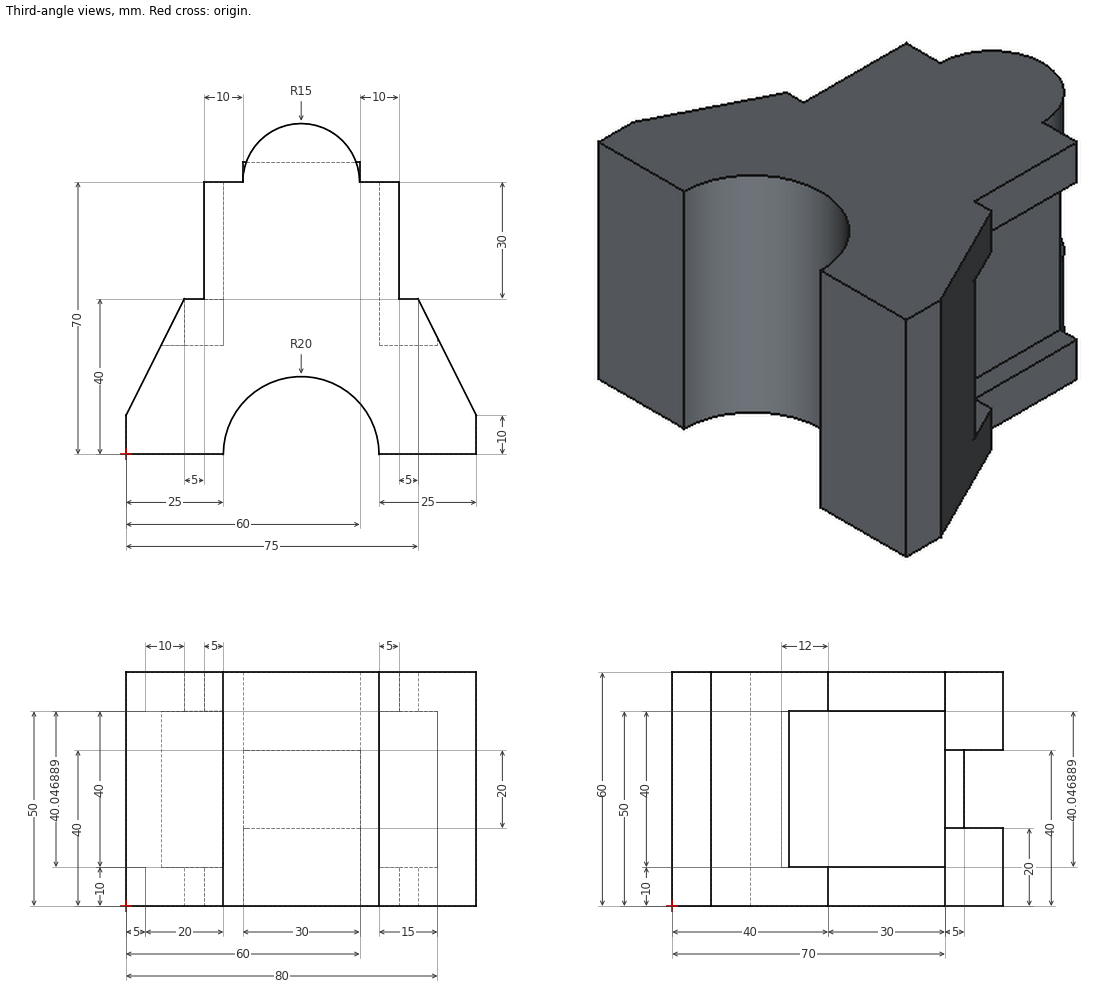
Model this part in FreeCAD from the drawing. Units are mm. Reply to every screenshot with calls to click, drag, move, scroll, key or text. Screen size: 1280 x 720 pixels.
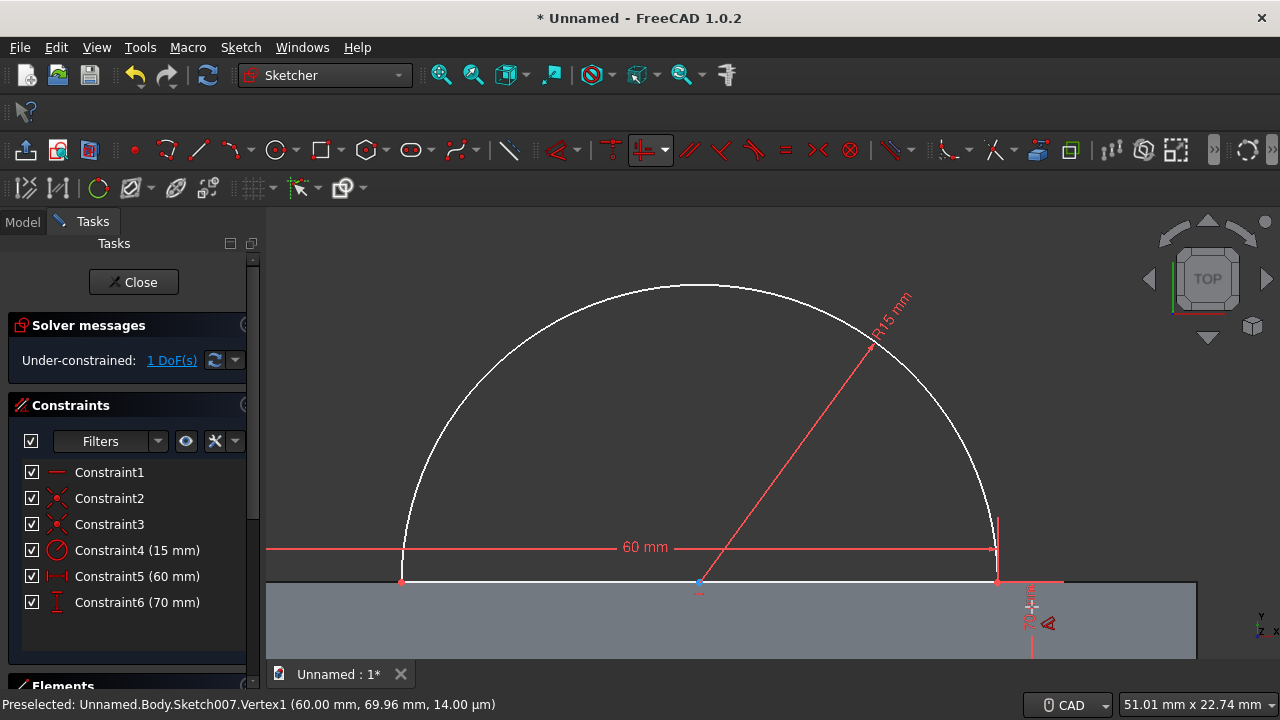
click(700, 583)
click(734, 607)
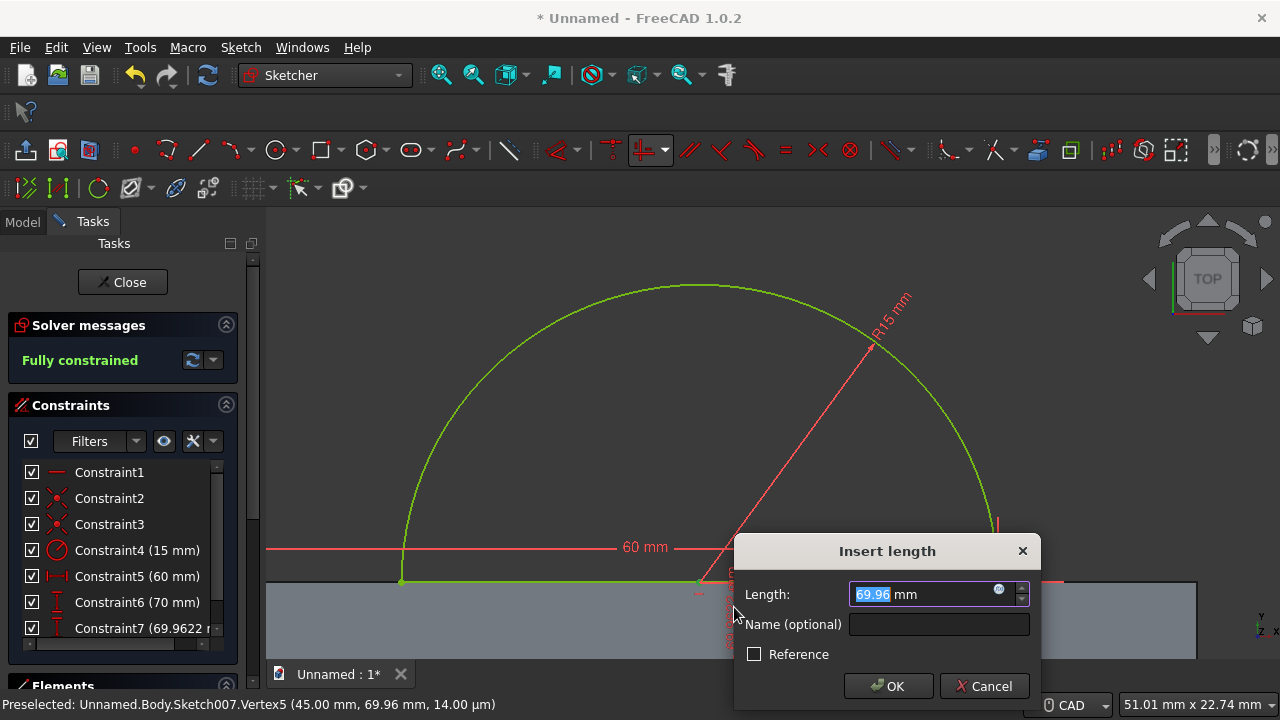
text(70)
key(Return)
key(Escape)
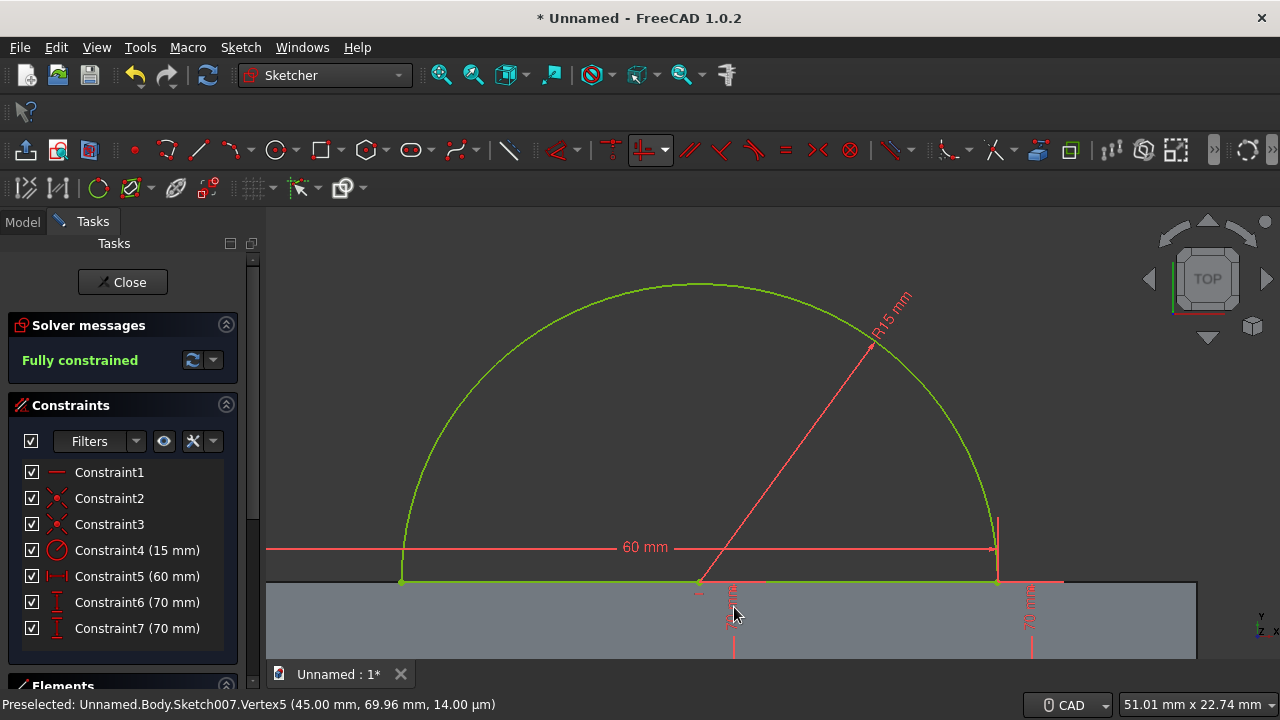
click(123, 282)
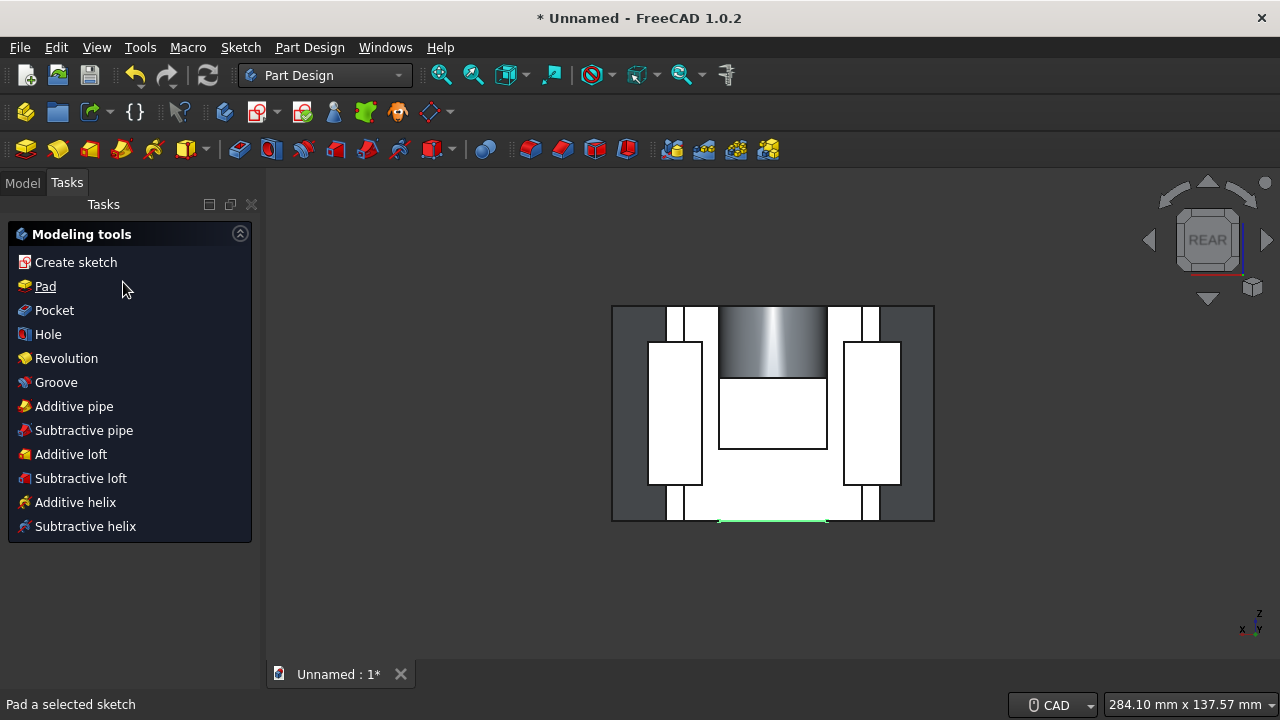
click(26, 150)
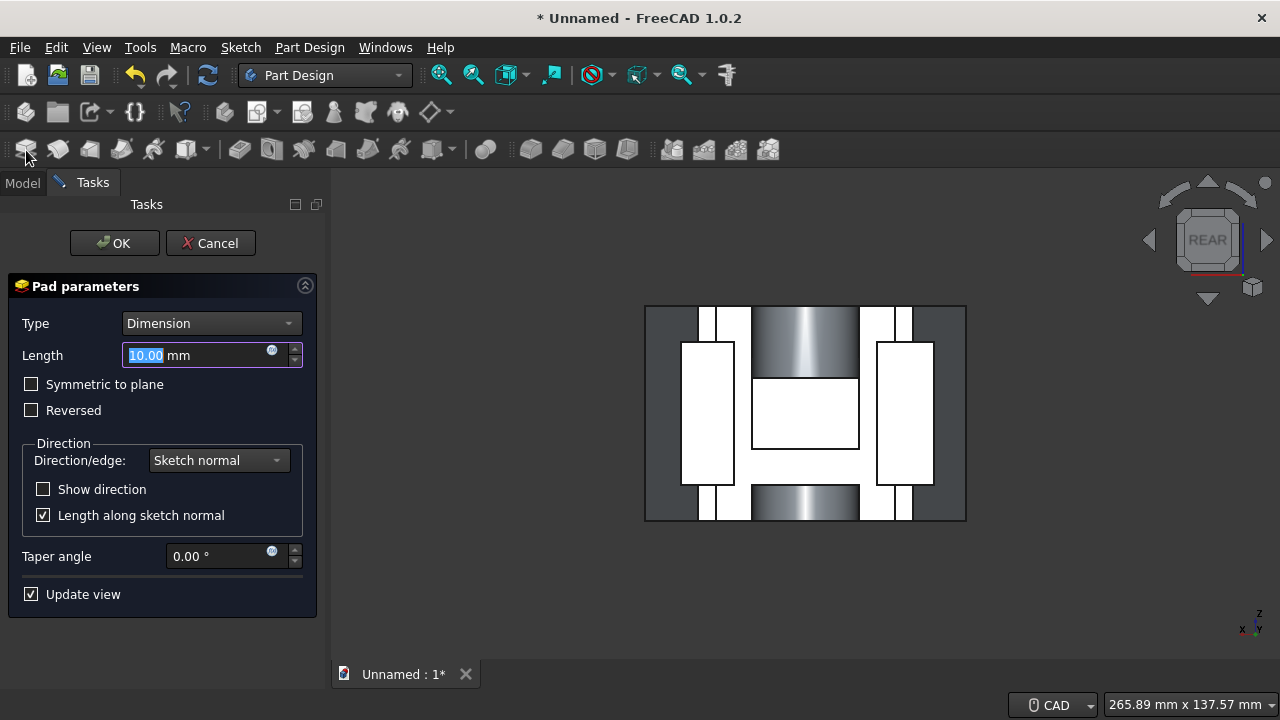
text(20)
key(Tab)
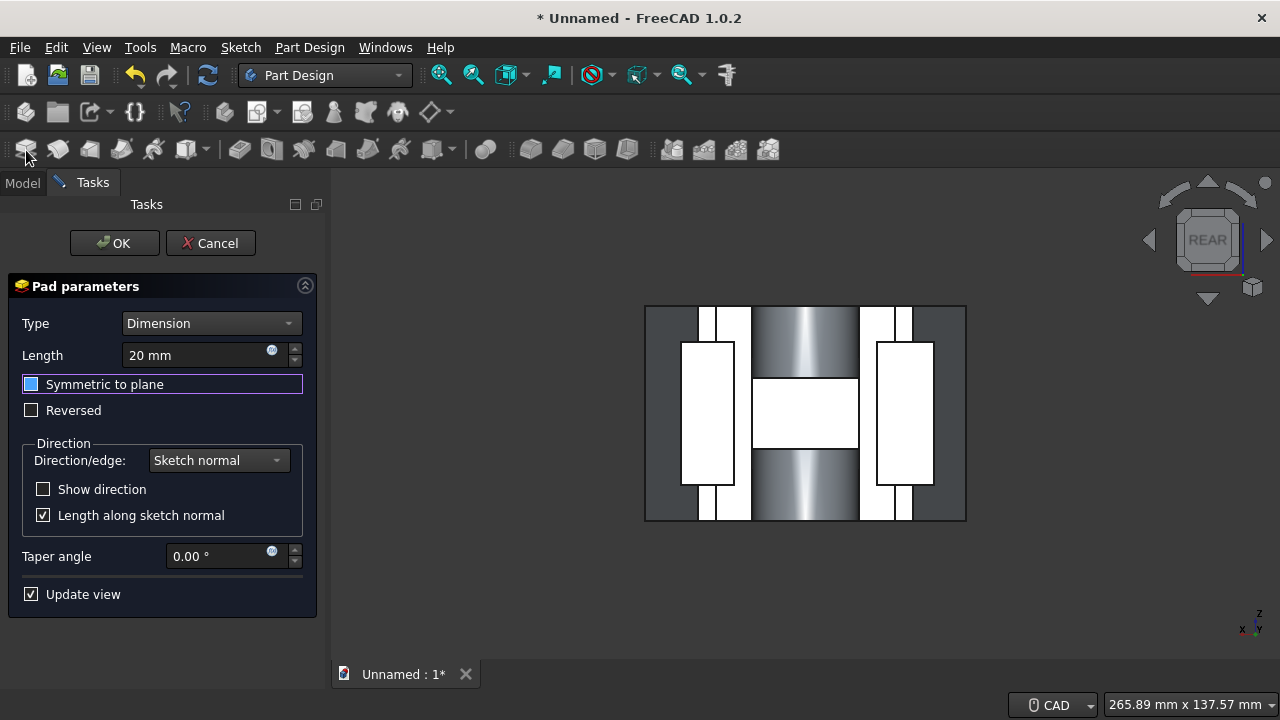
click(115, 243)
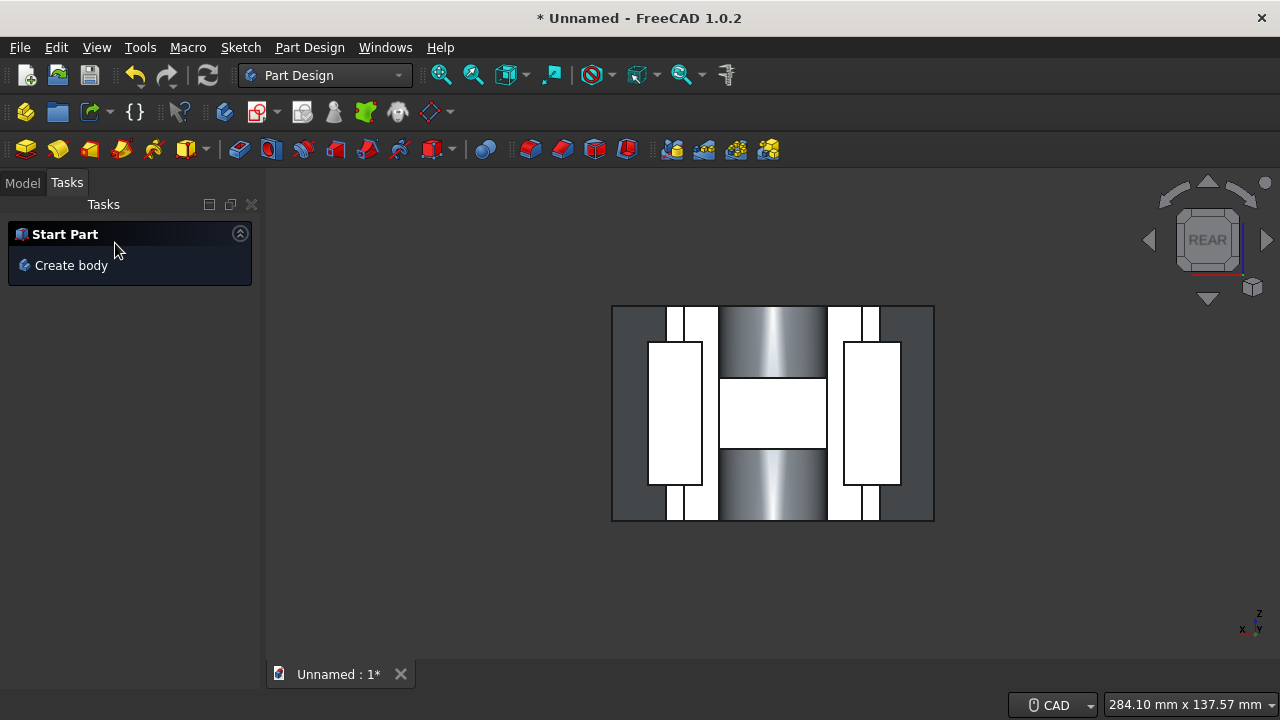
key(0)